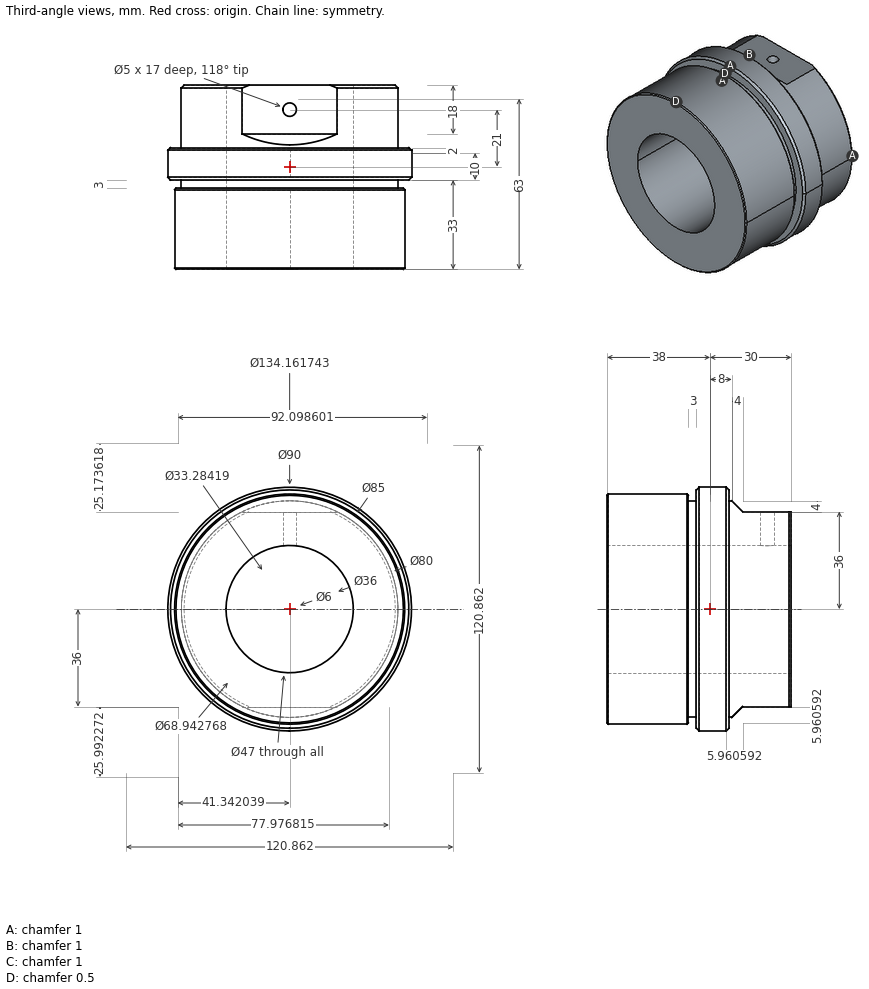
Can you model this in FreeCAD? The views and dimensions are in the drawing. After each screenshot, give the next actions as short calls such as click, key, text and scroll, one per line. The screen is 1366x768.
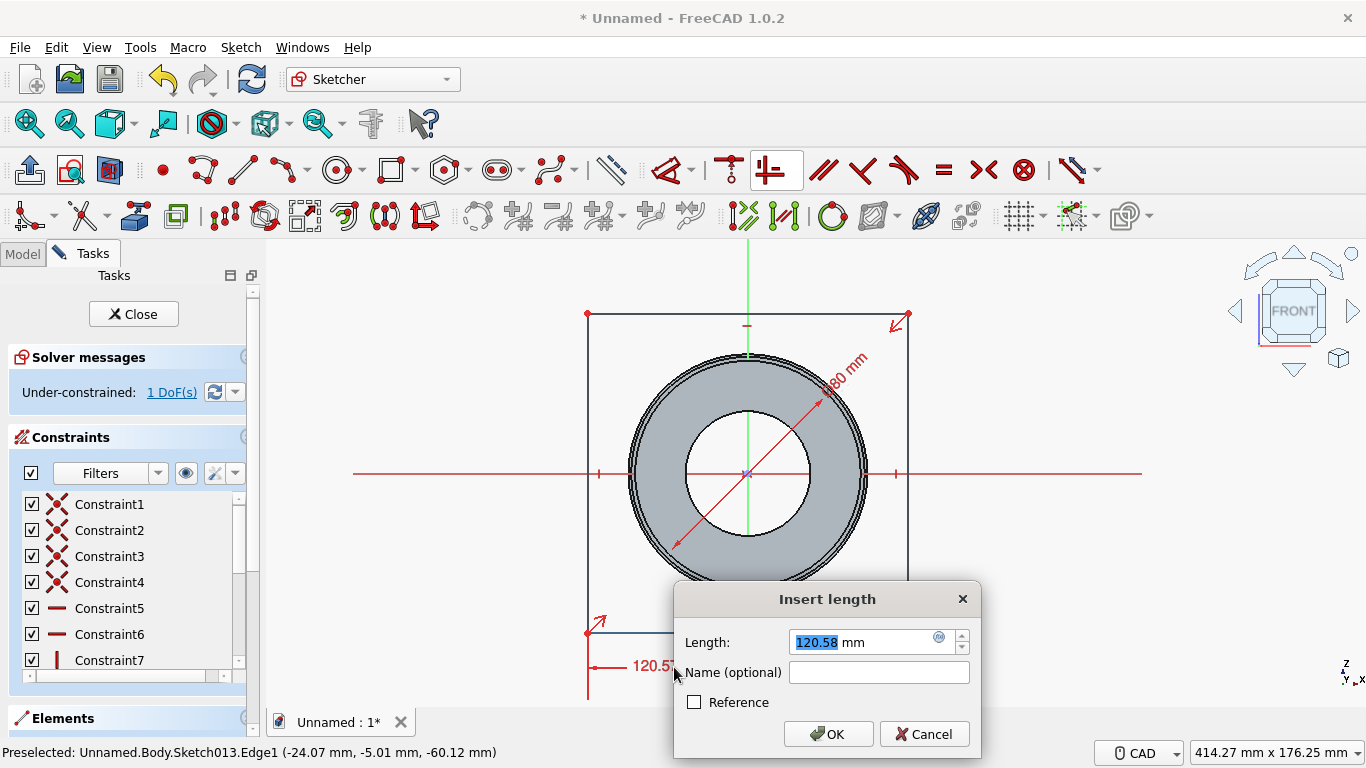
text(120.862)
key(Return)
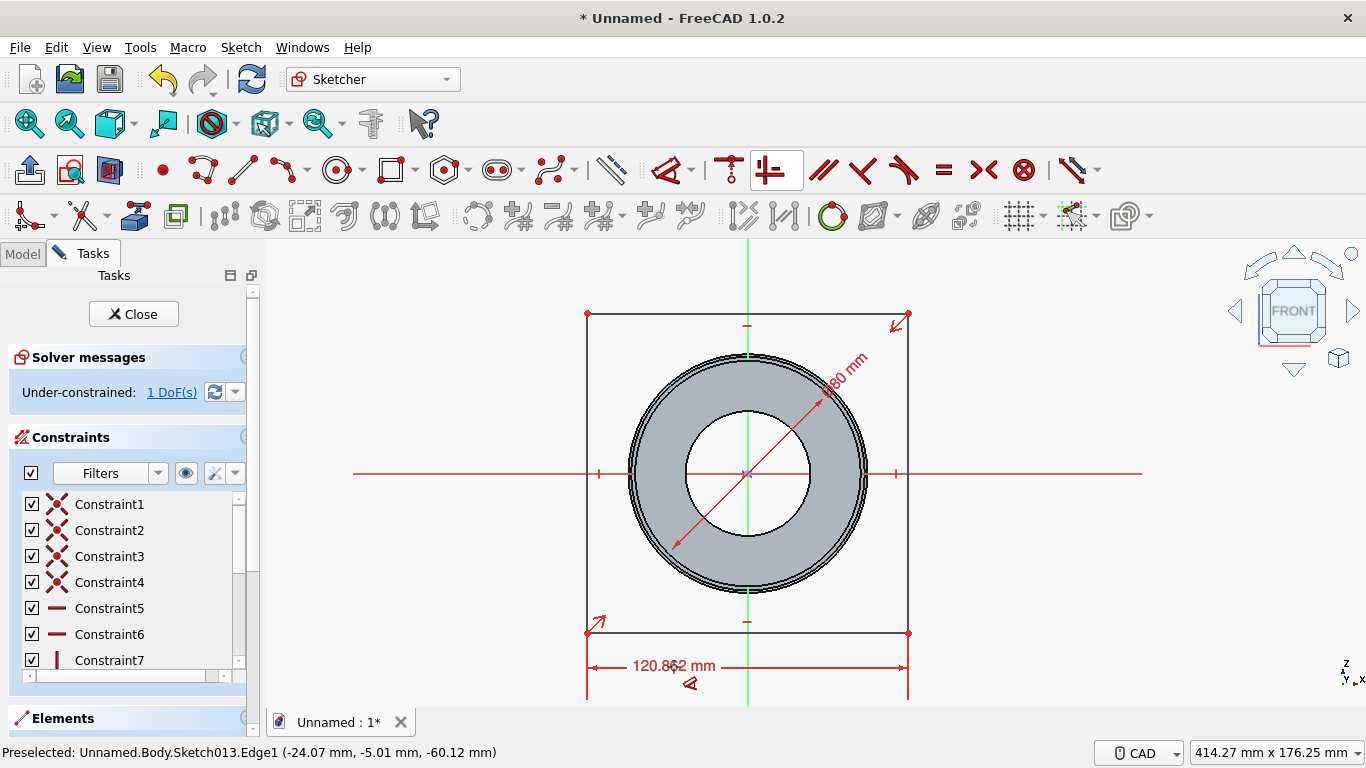
click(908, 537)
click(942, 400)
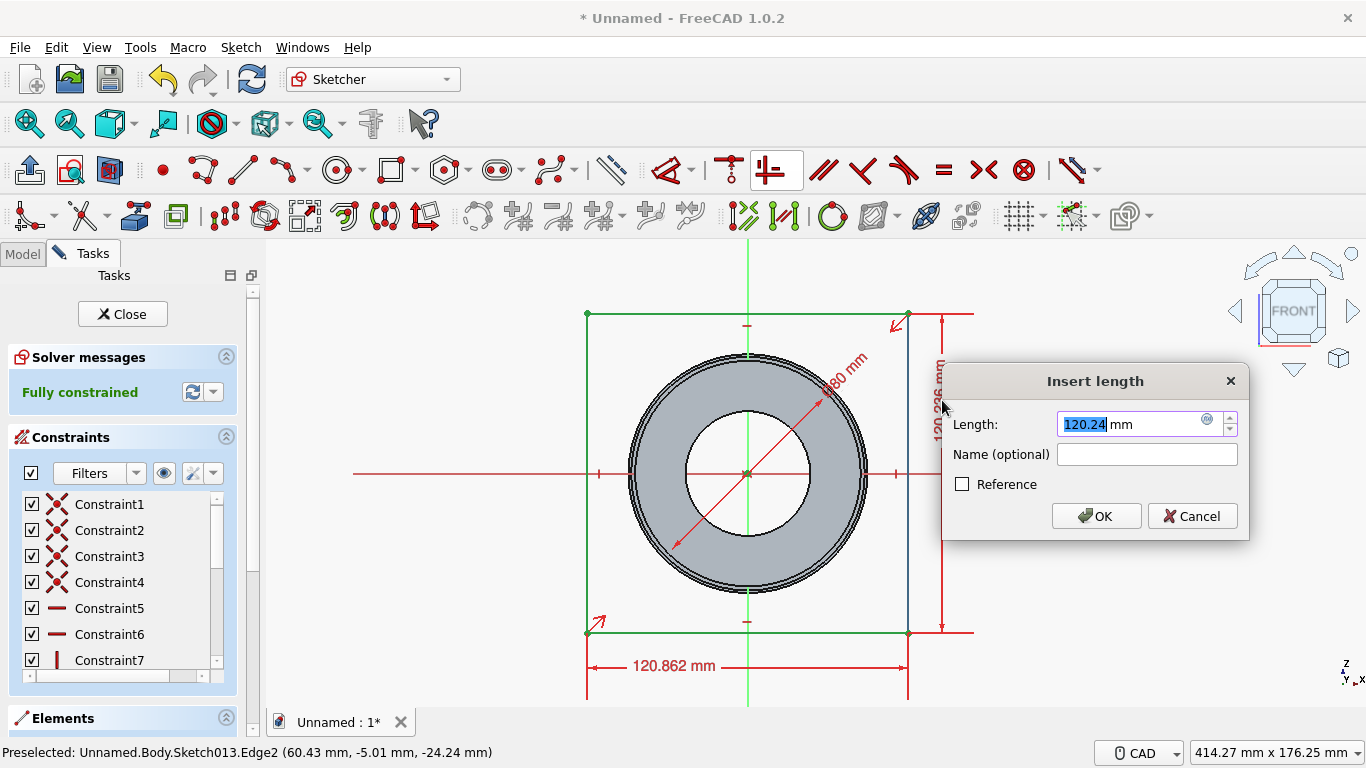
text(120.862)
key(Return)
key(Escape)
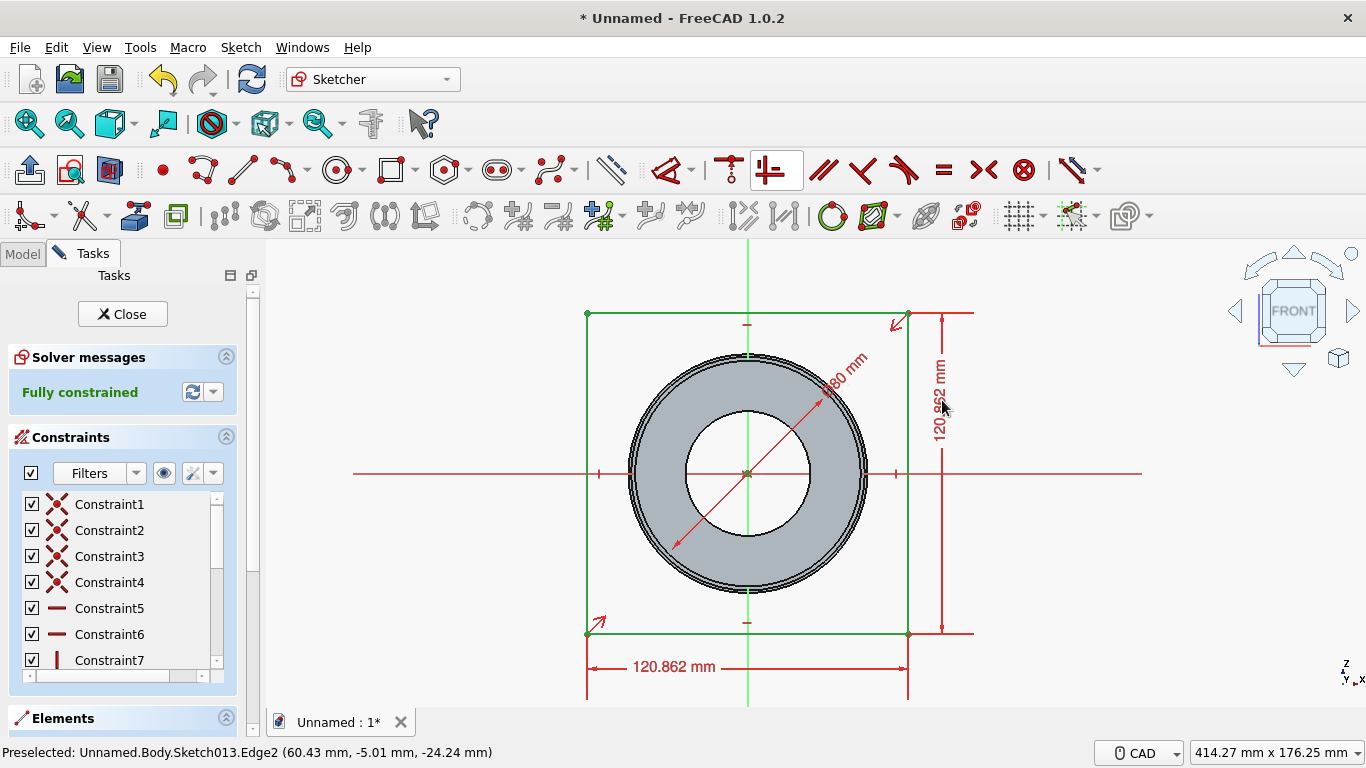
click(123, 314)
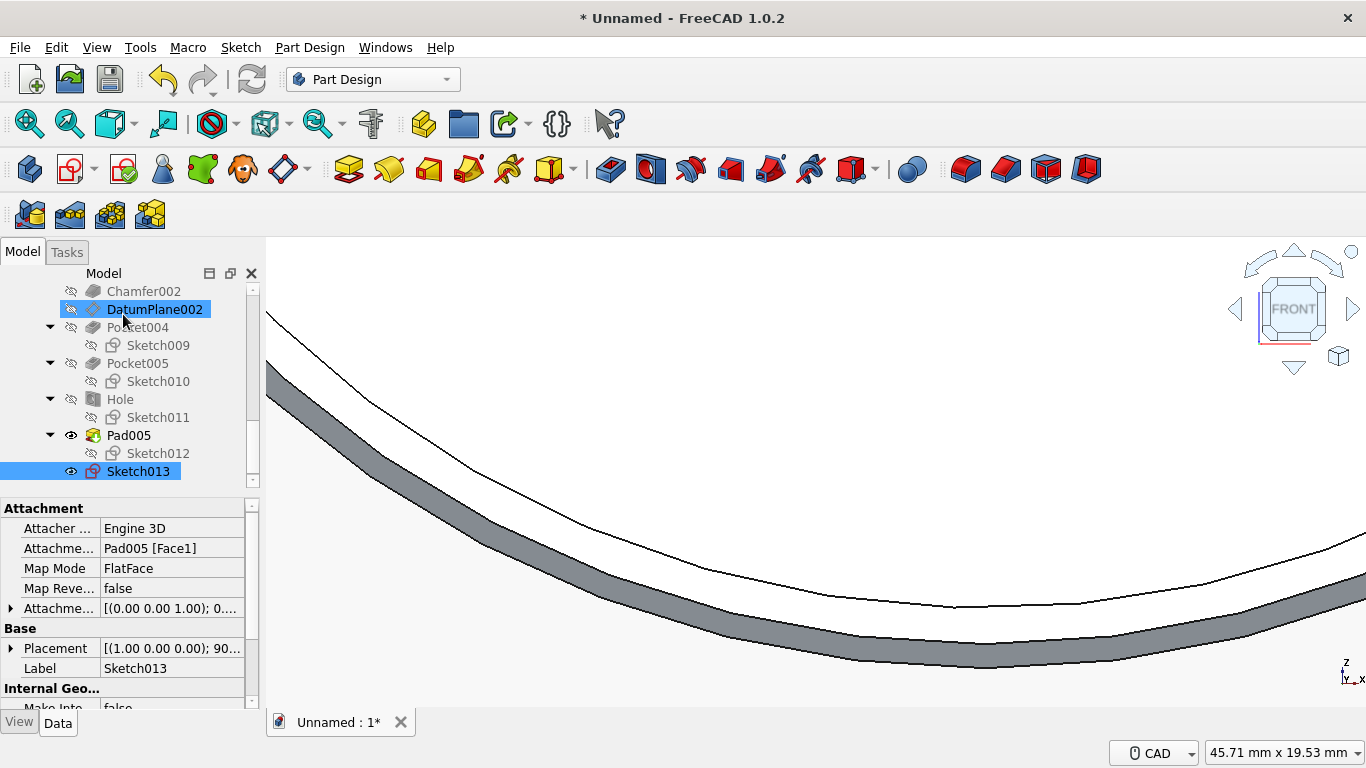
click(612, 170)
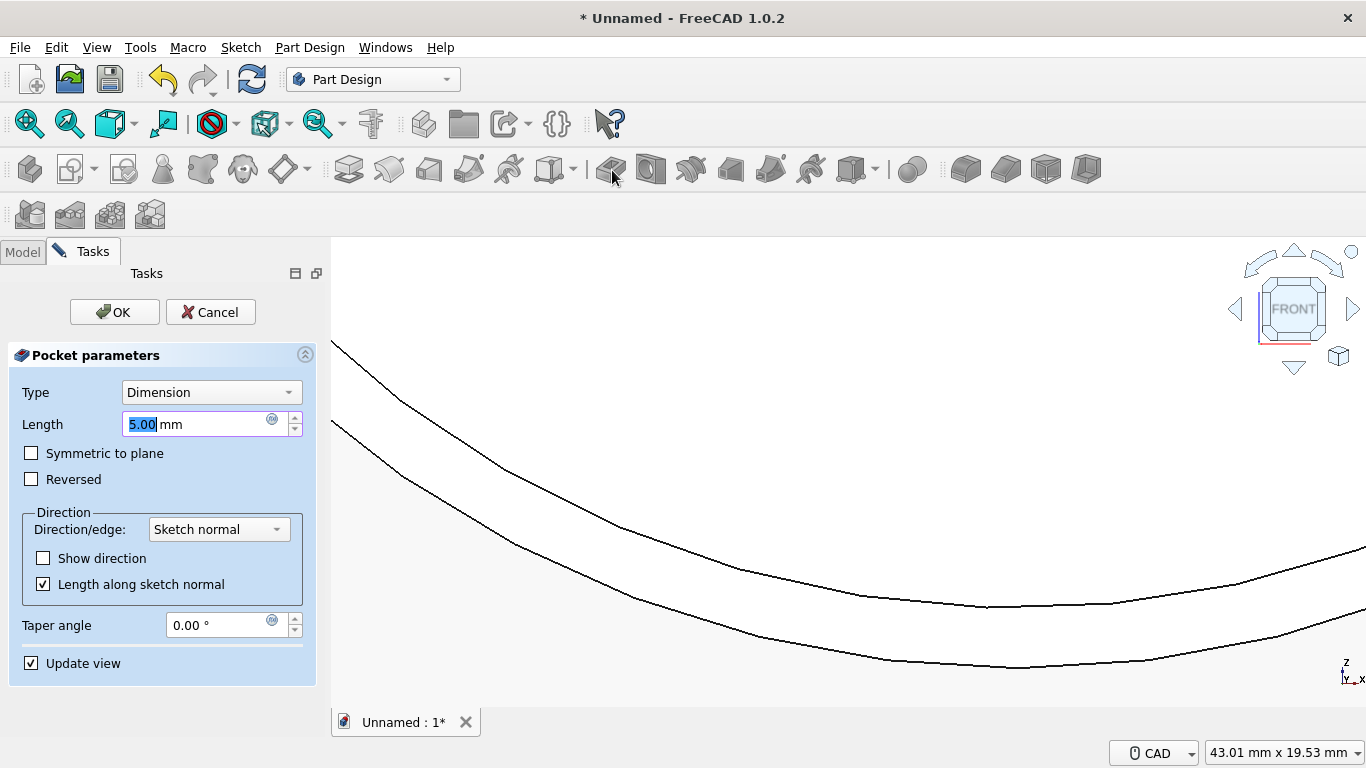
text(3)
key(Tab)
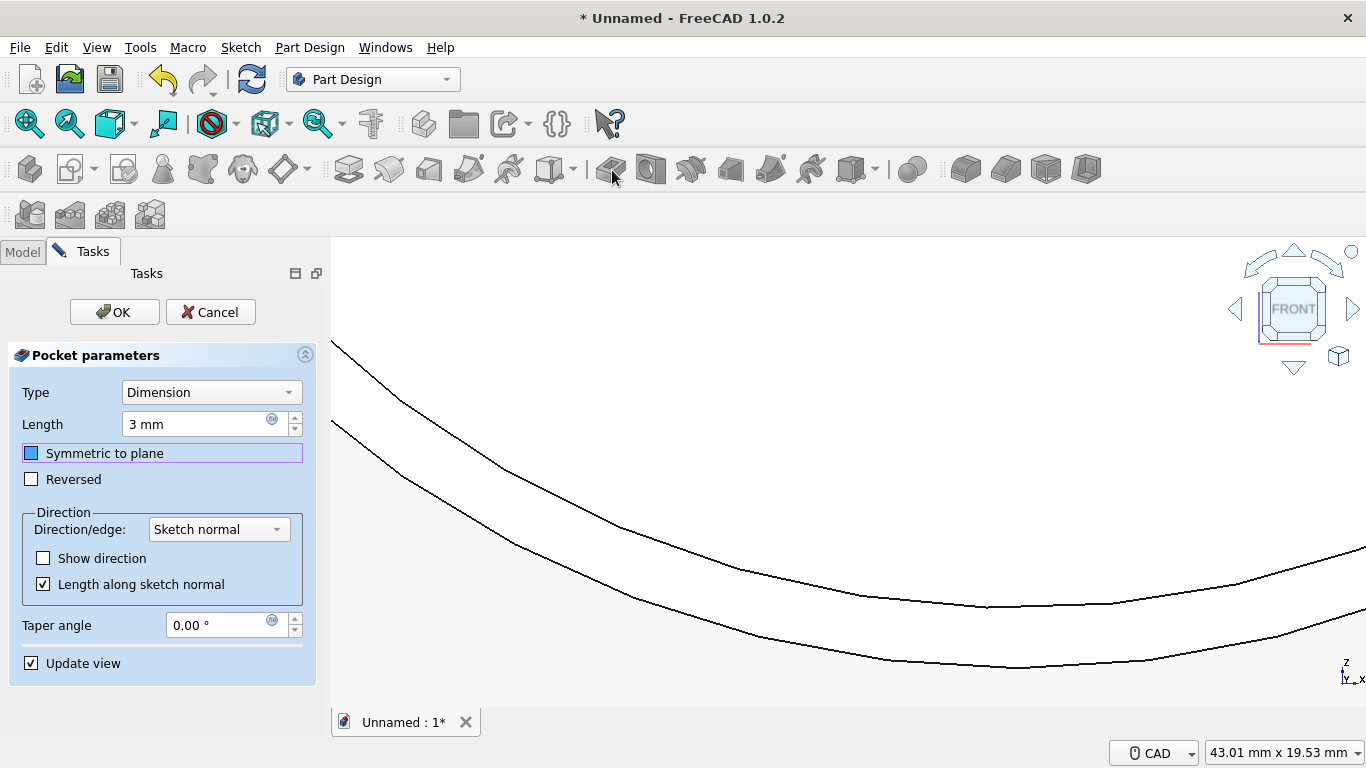
click(30, 479)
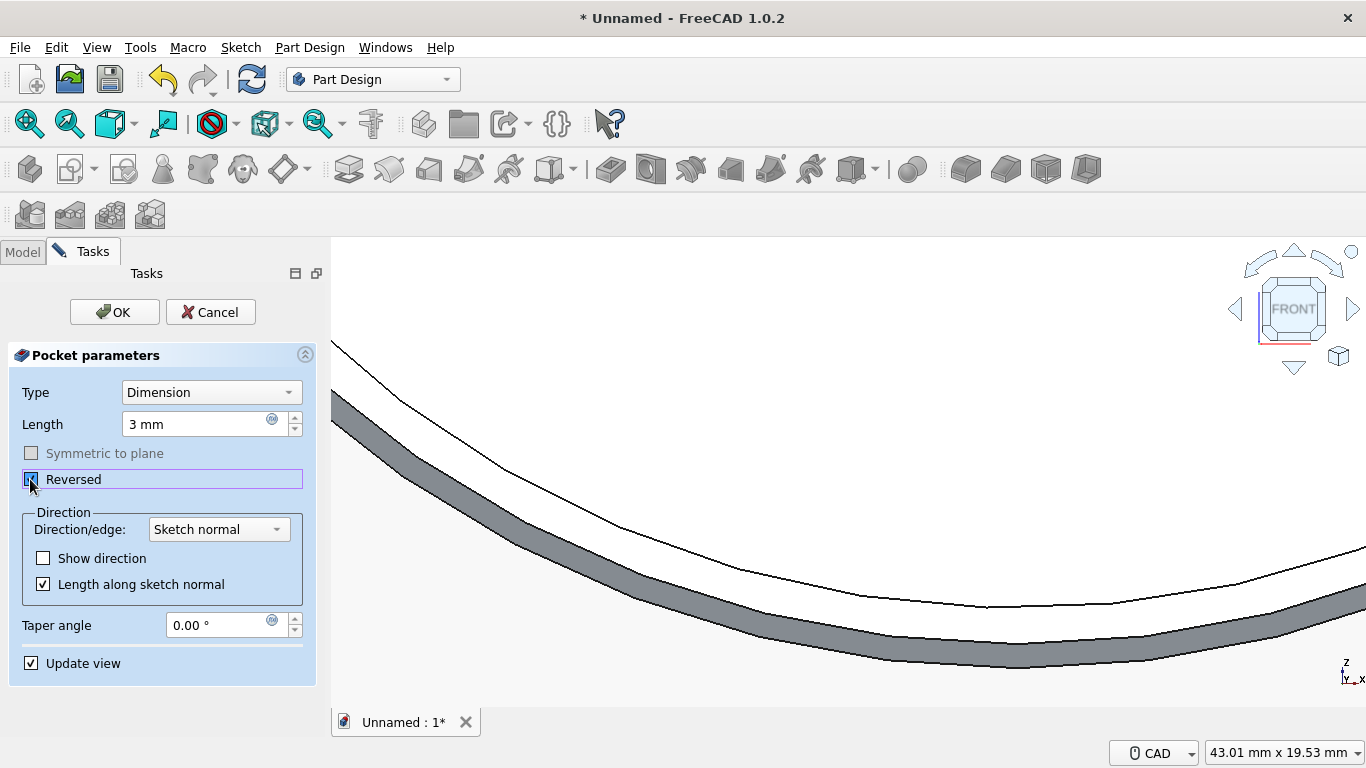
click(115, 312)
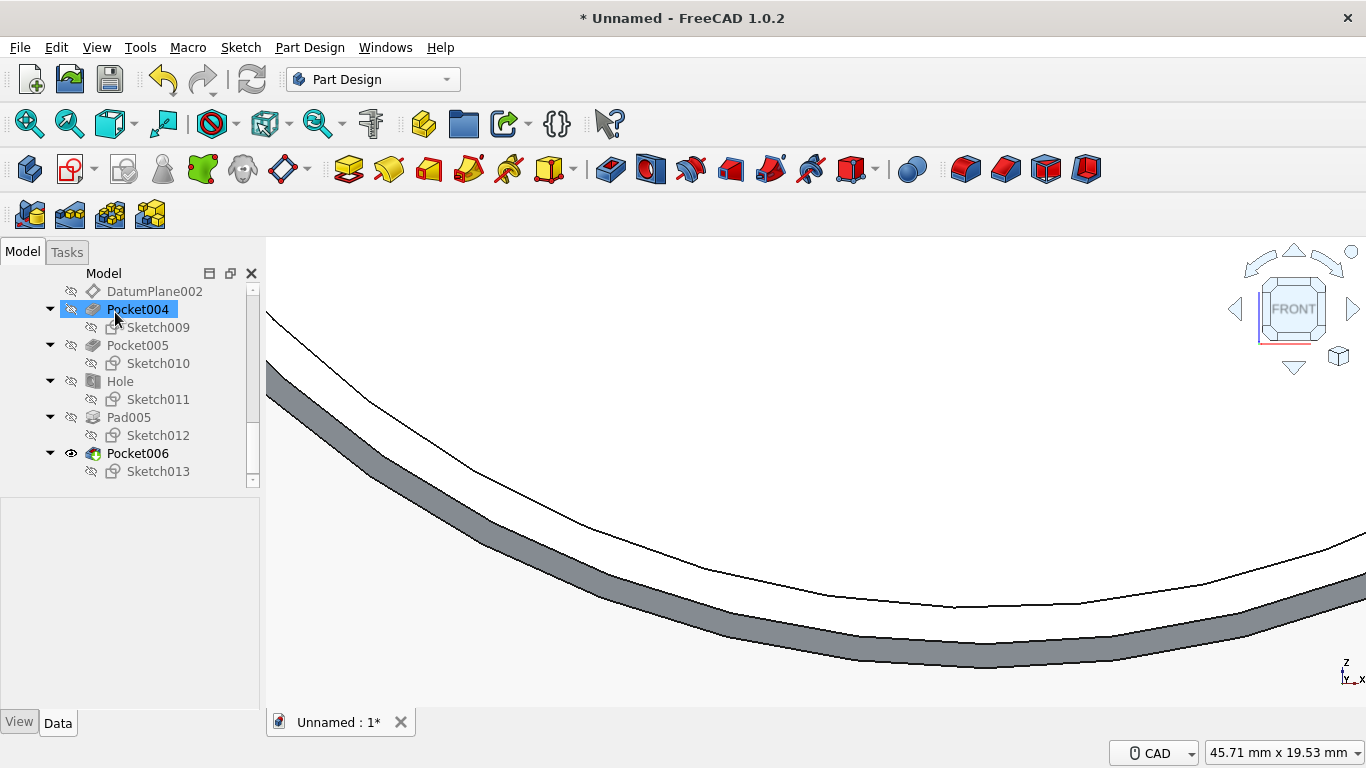
click(30, 124)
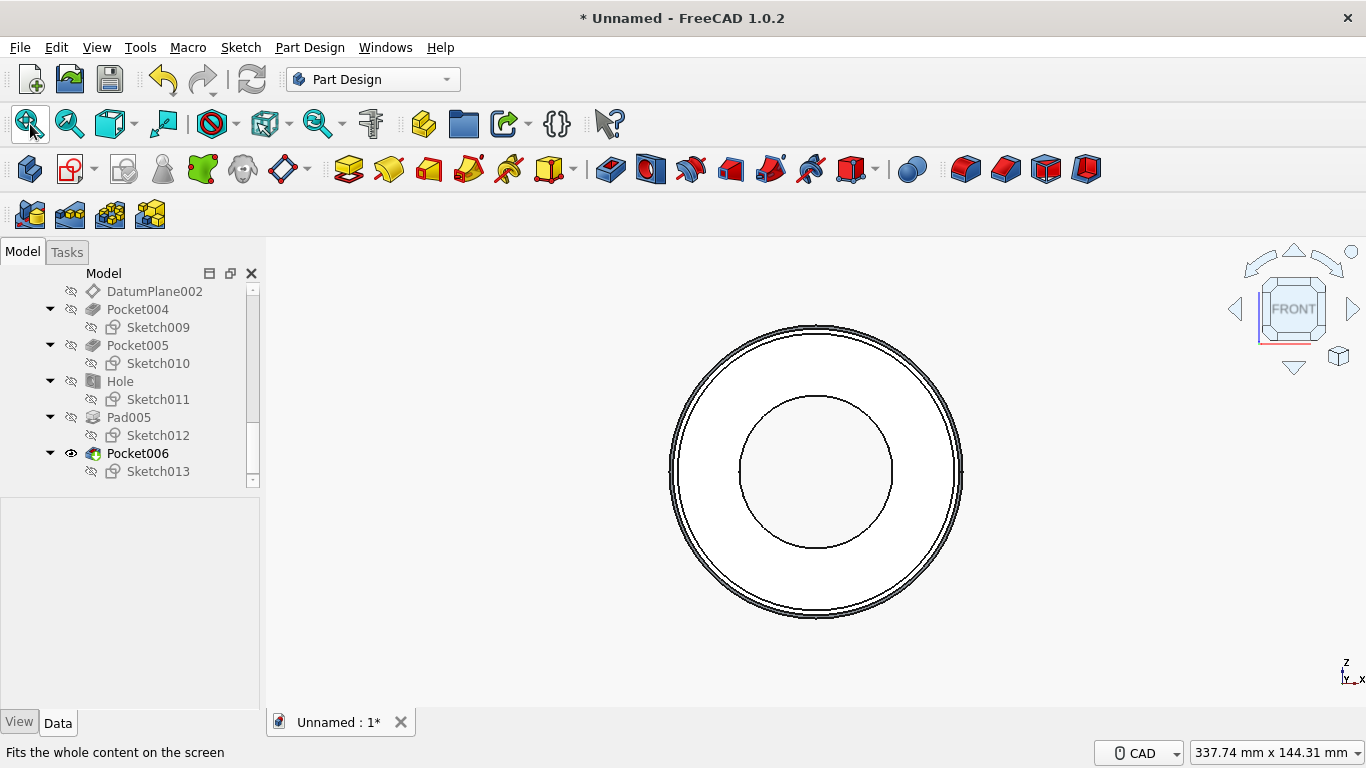
click(678, 471)